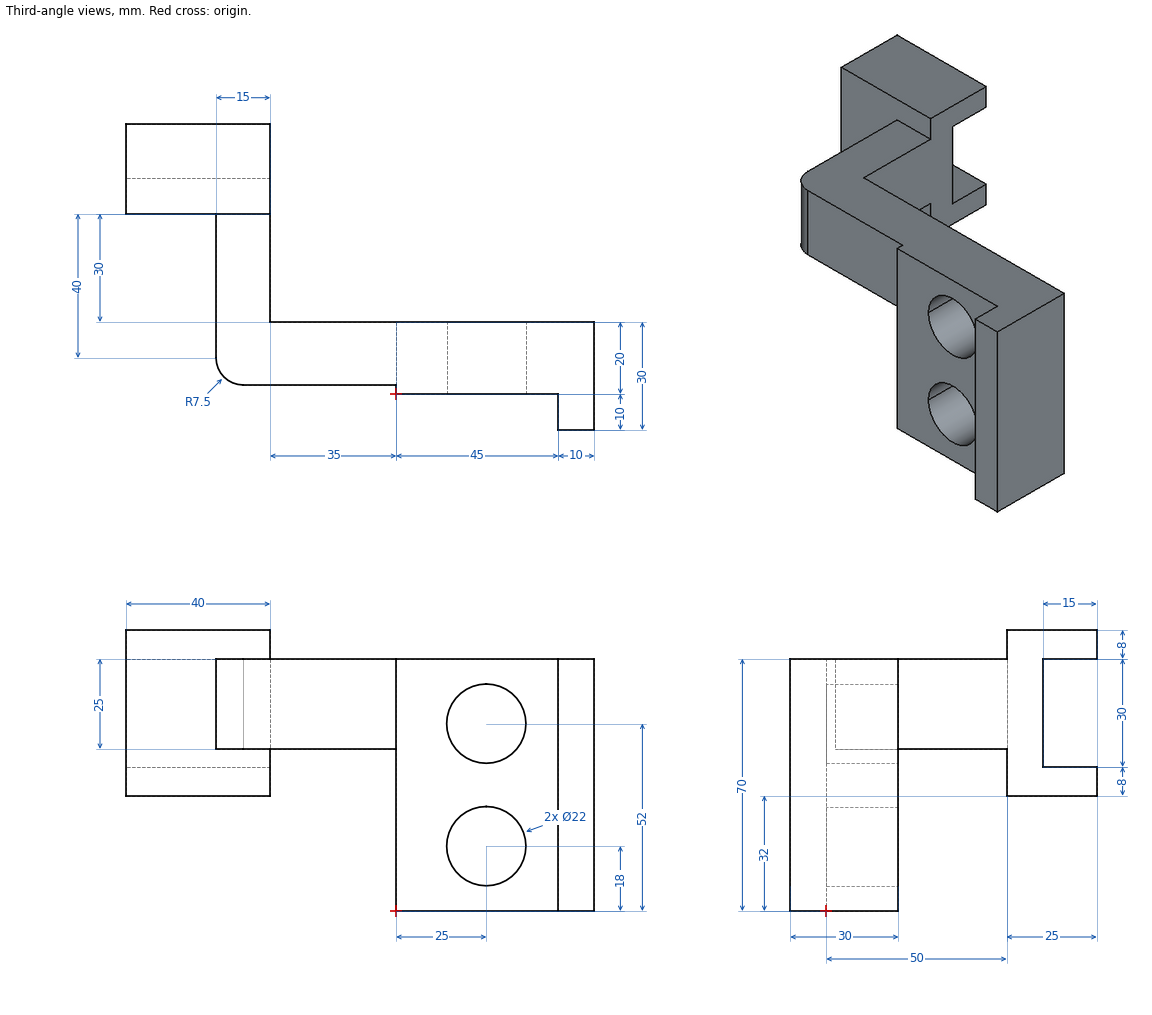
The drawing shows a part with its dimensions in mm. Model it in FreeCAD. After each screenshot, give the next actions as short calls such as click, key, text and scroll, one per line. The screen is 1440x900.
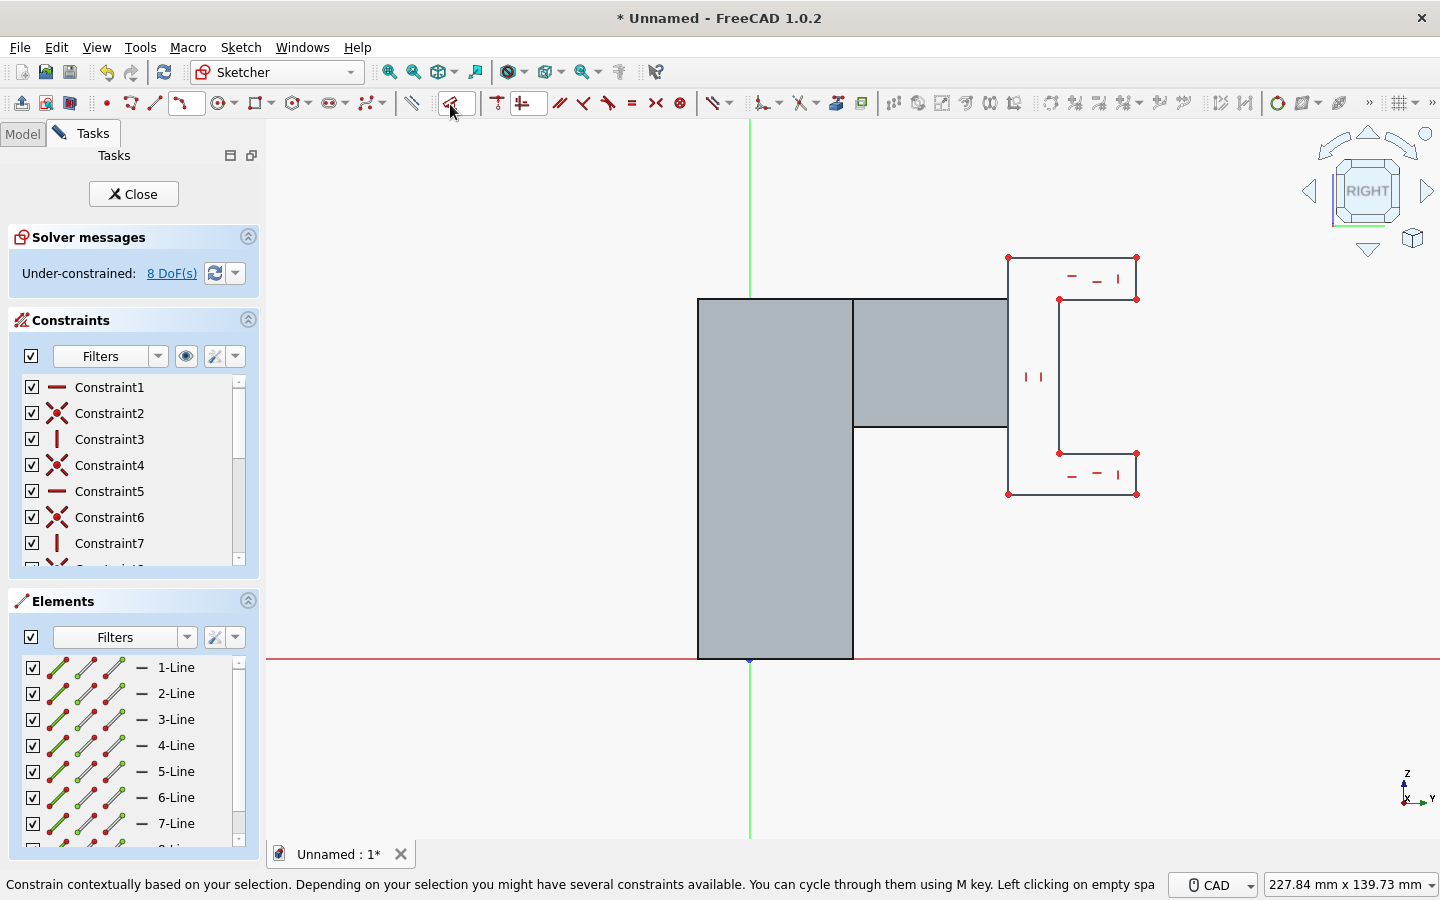
click(1136, 483)
click(1170, 475)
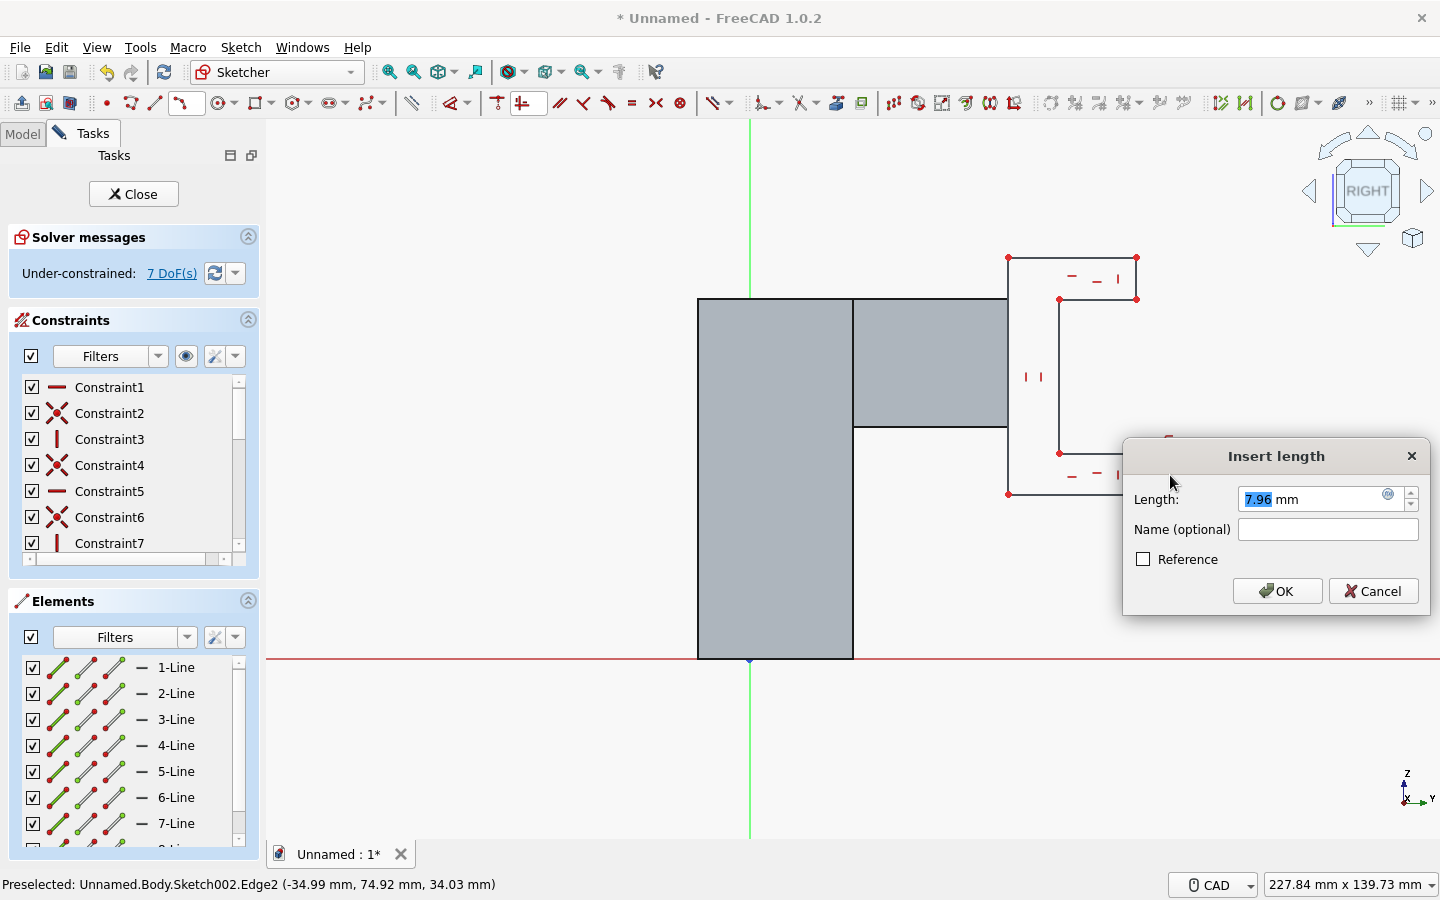
text(8)
key(Return)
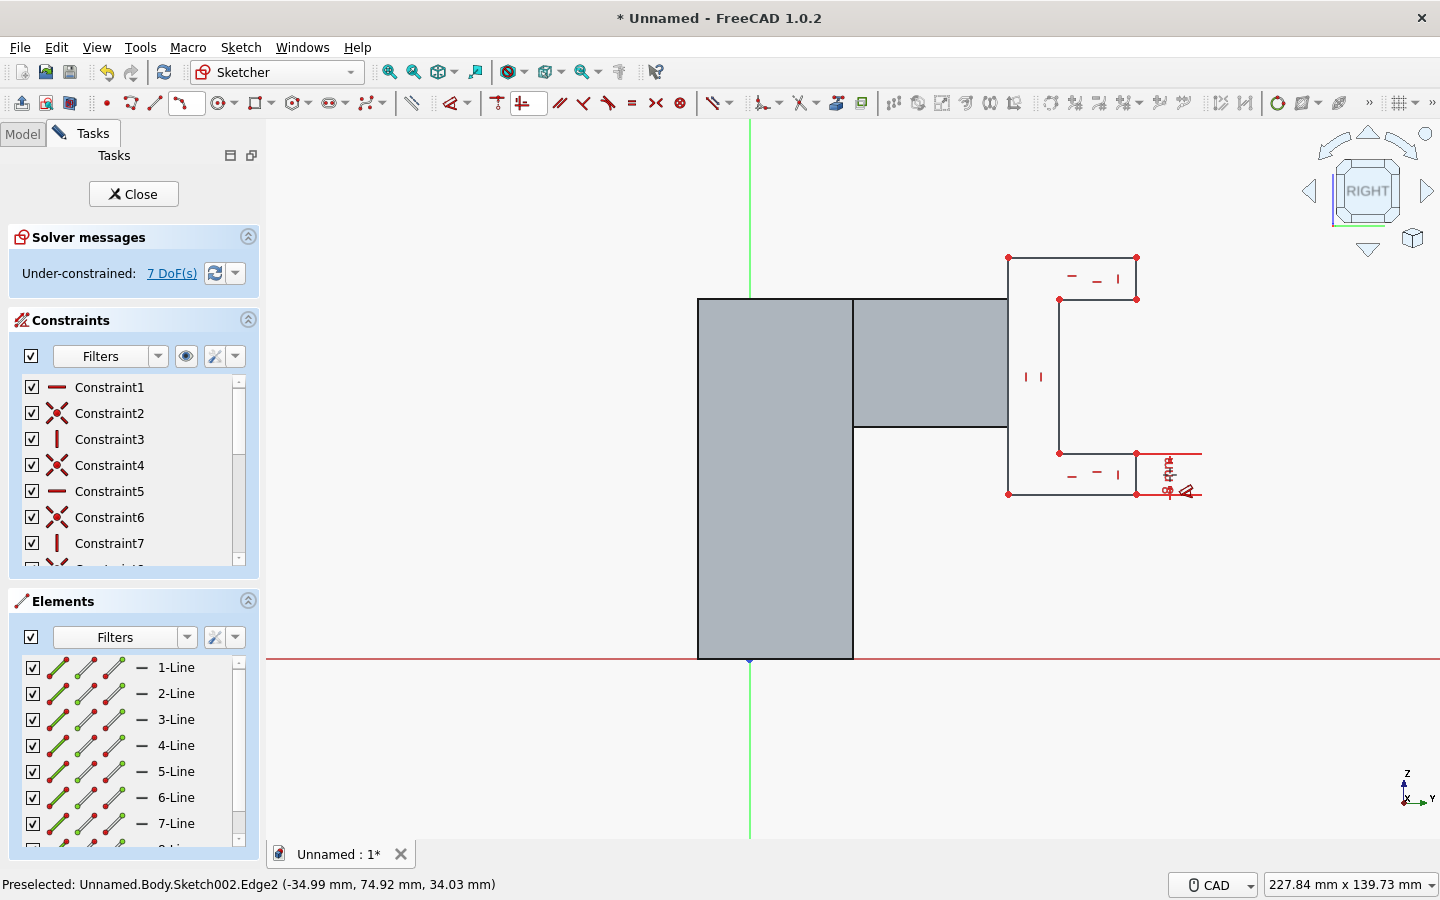
click(1136, 287)
click(1170, 279)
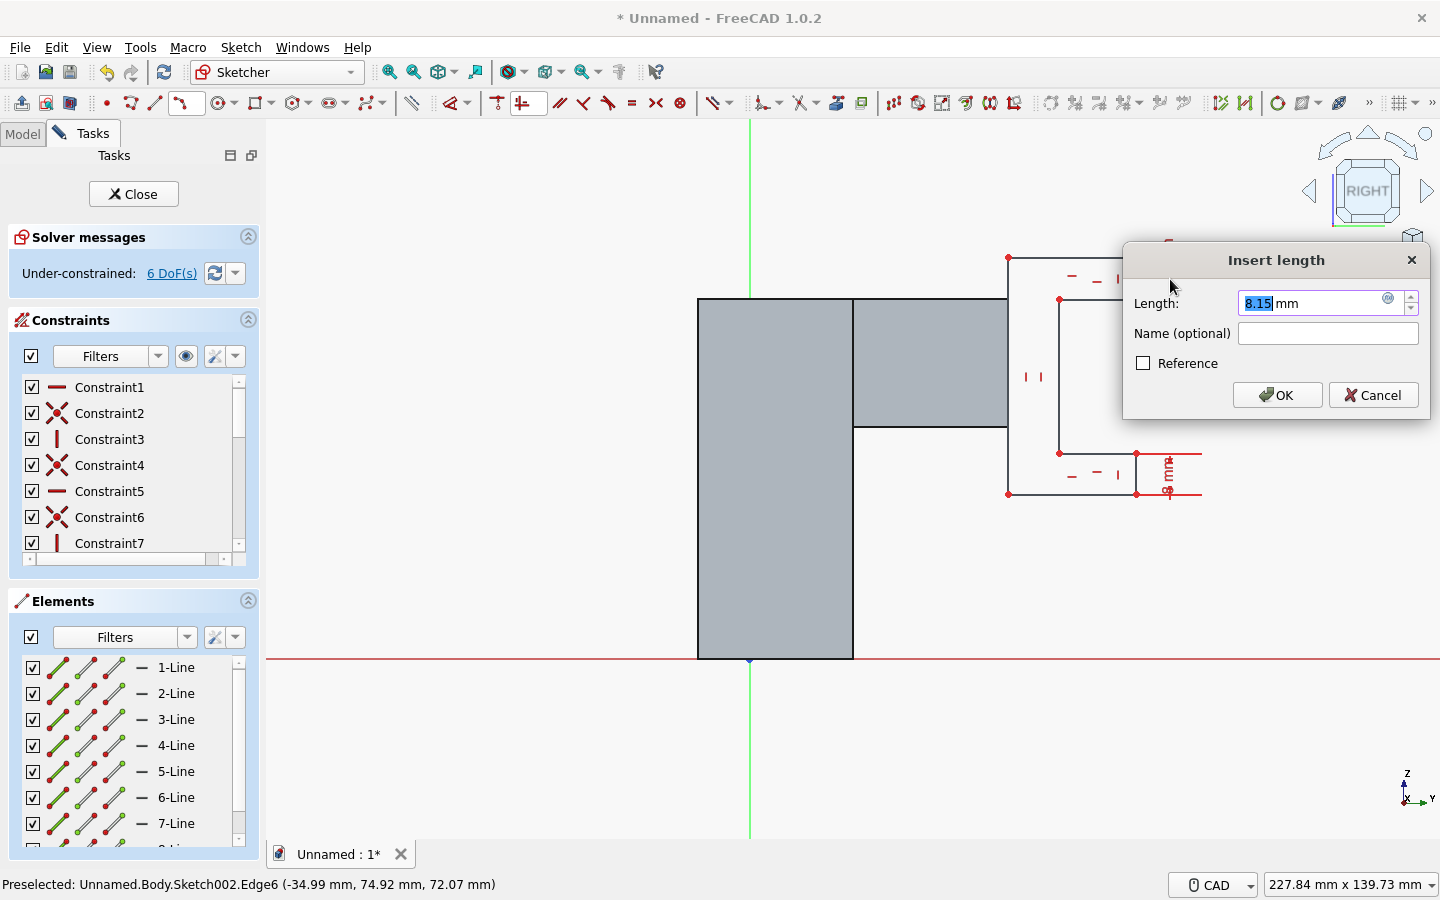
text(8)
key(Return)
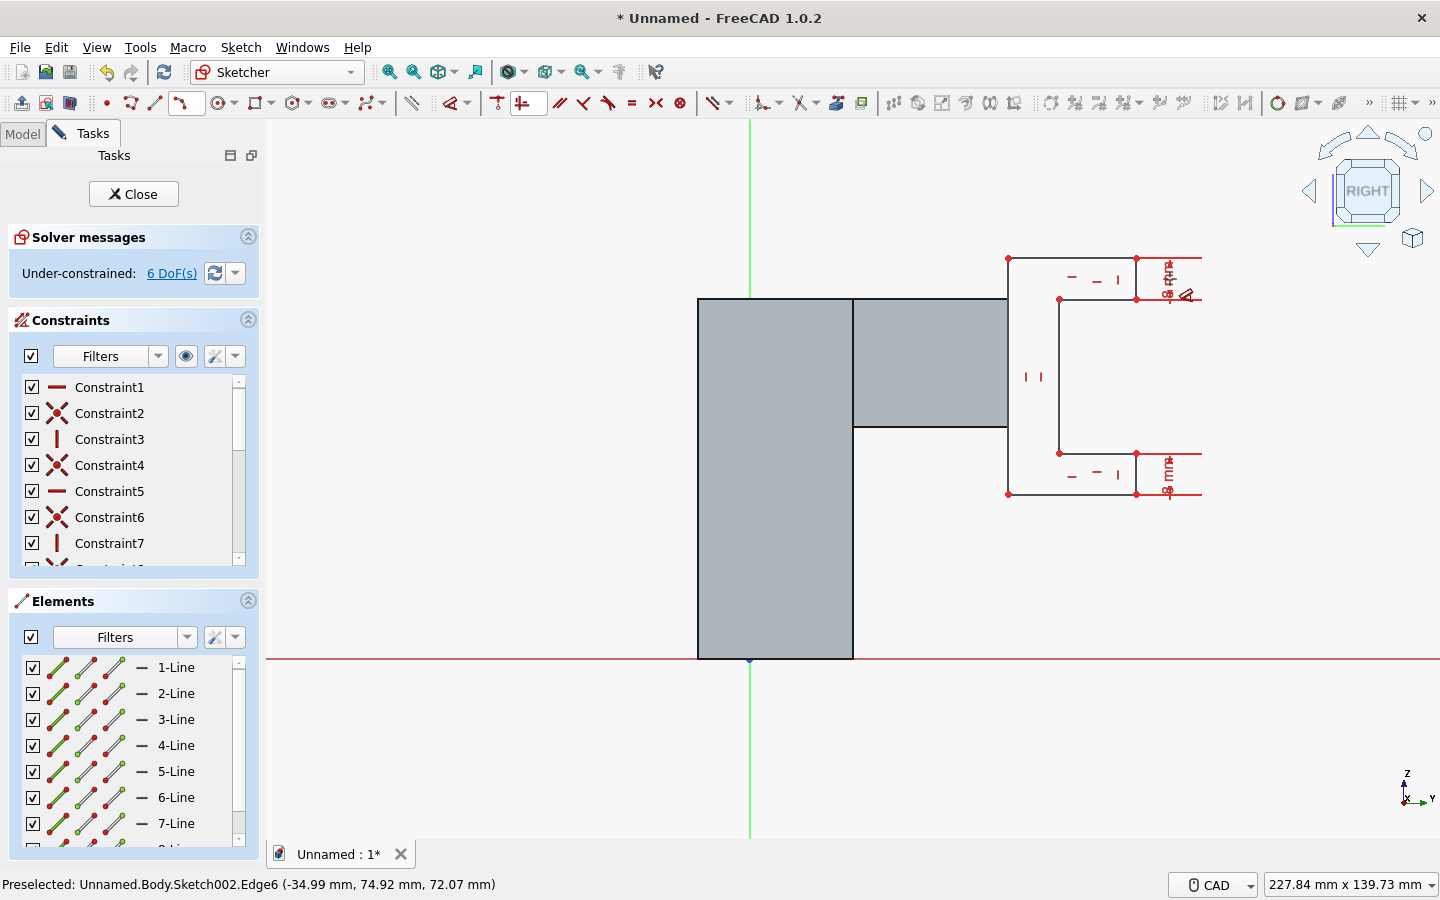
click(1046, 495)
click(1072, 529)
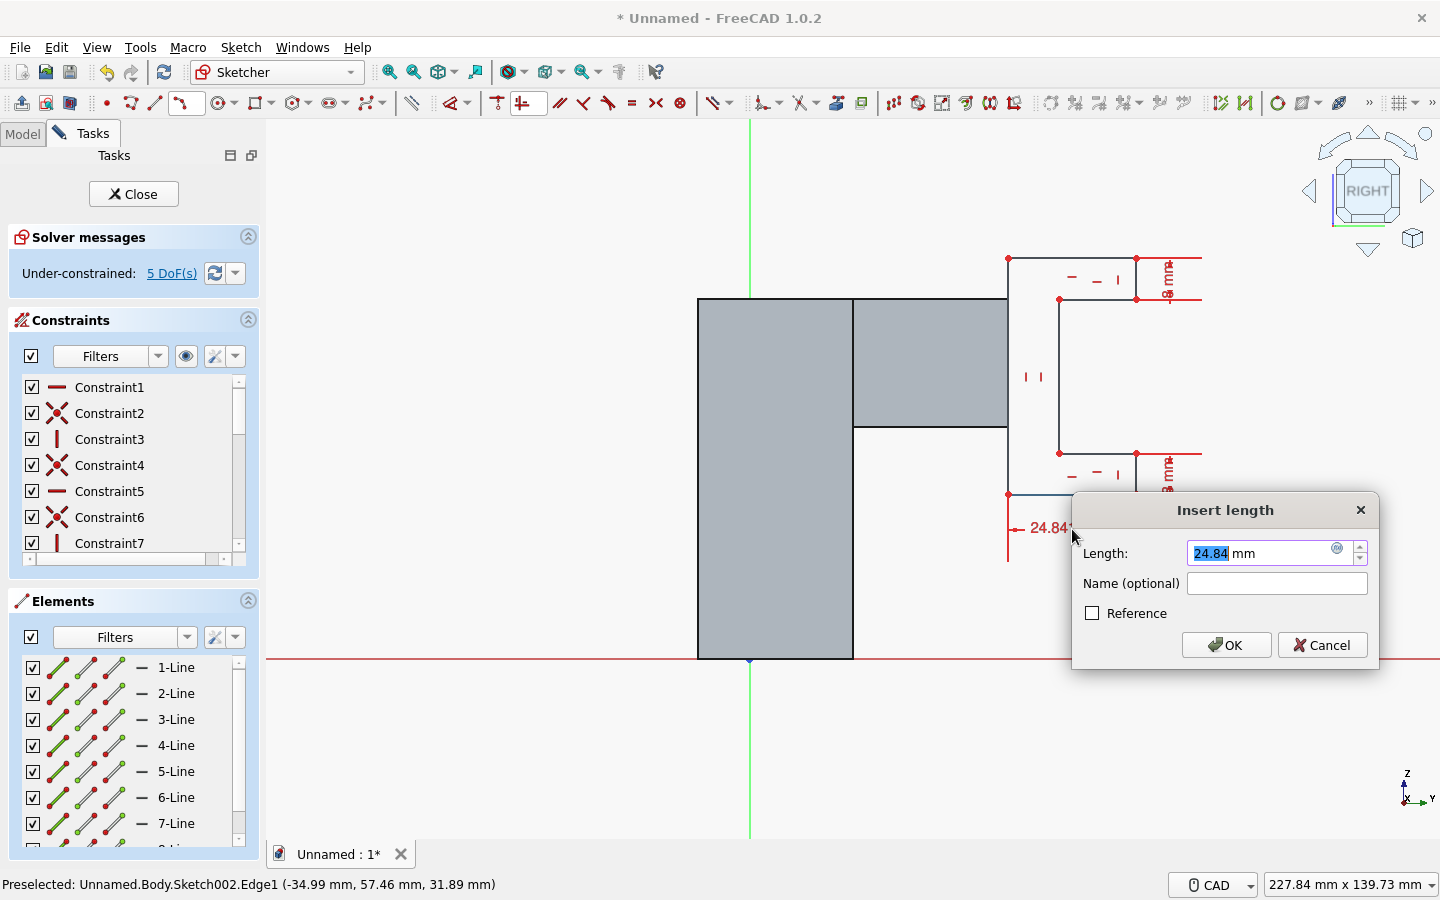
text(25)
key(Return)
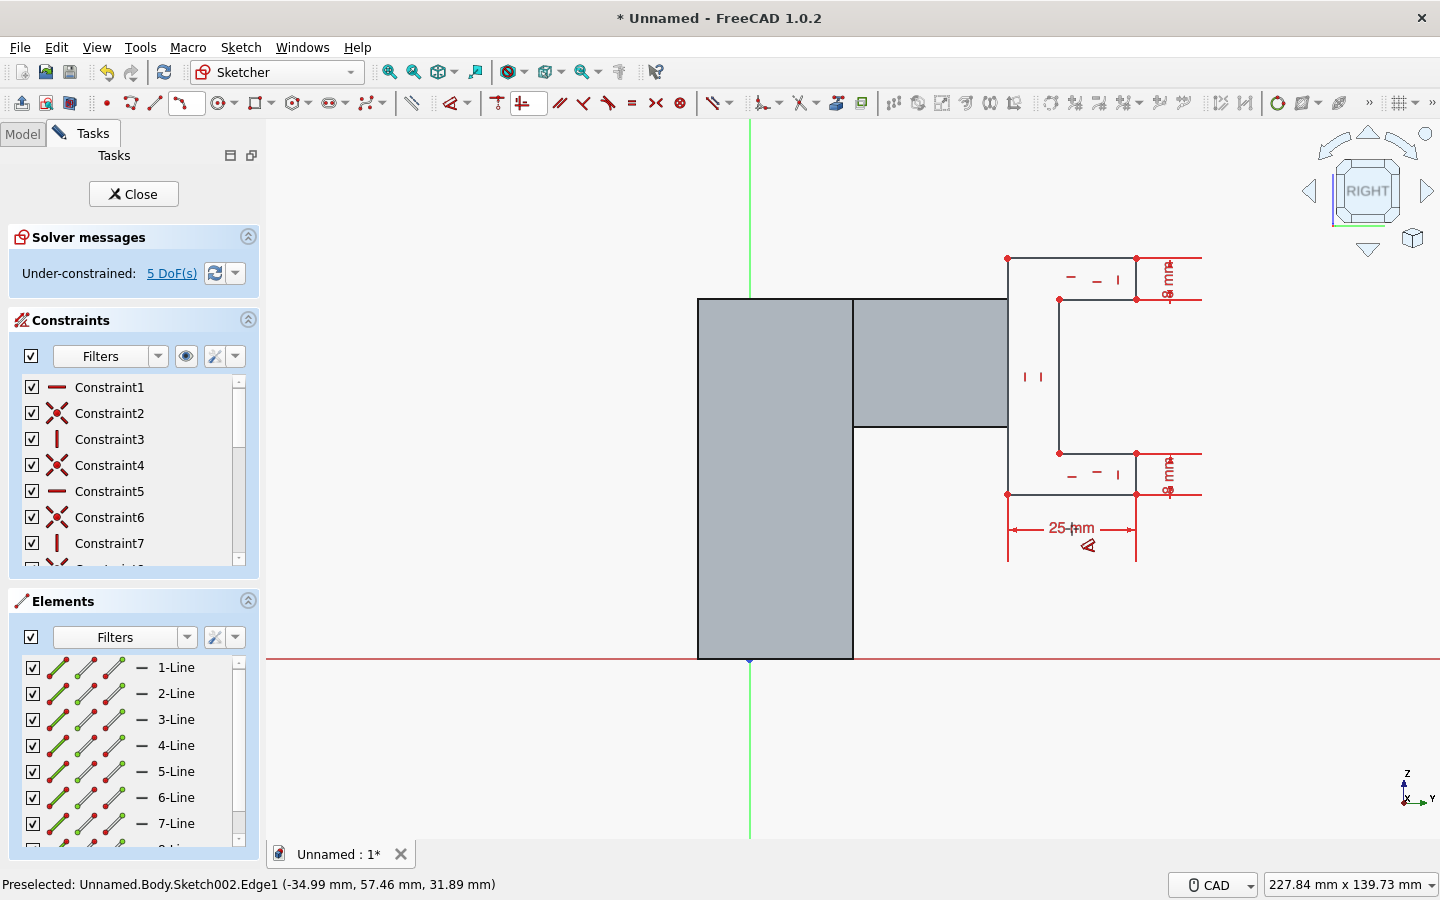
click(1113, 454)
click(1098, 420)